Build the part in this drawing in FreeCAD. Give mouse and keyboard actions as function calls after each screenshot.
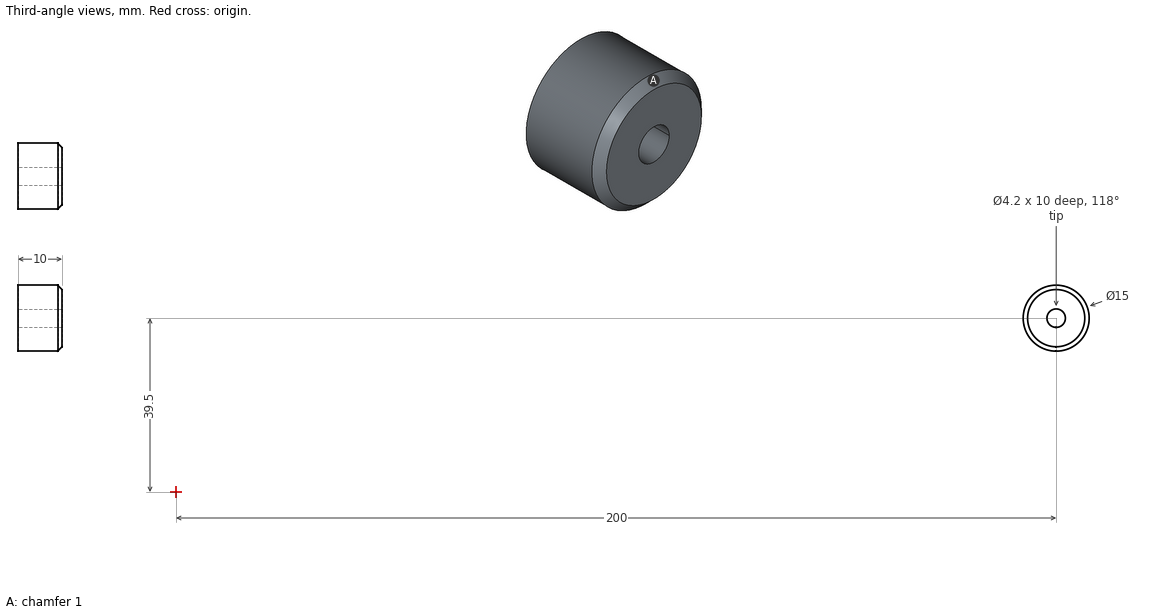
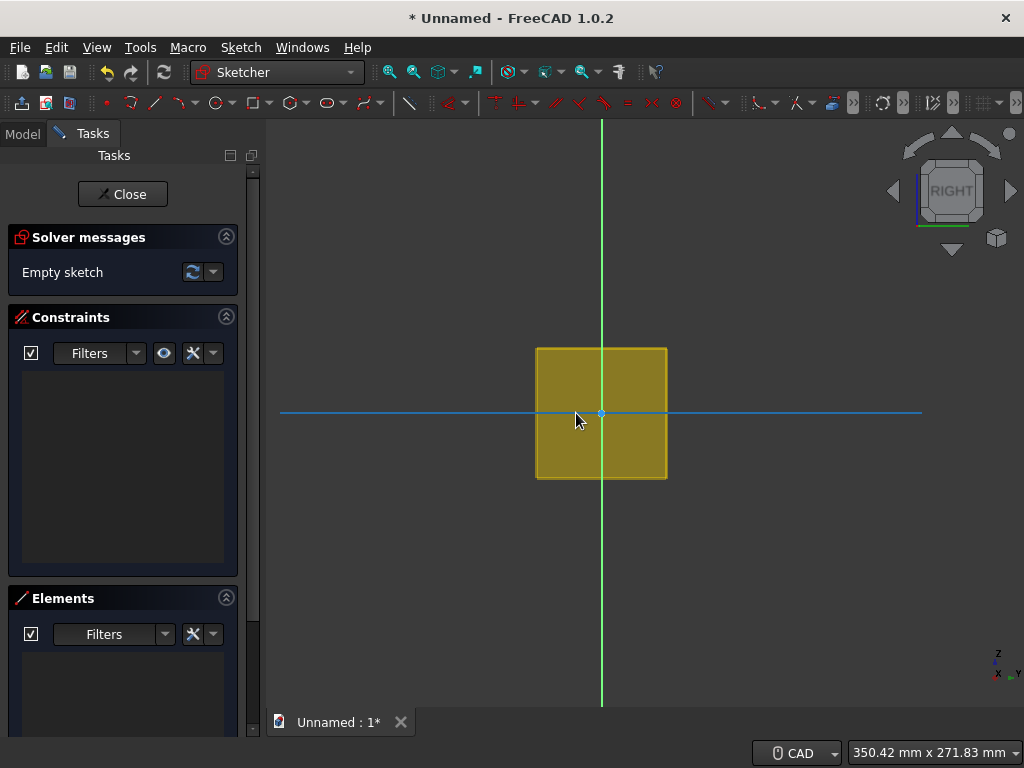
scroll(576, 413, down, 5)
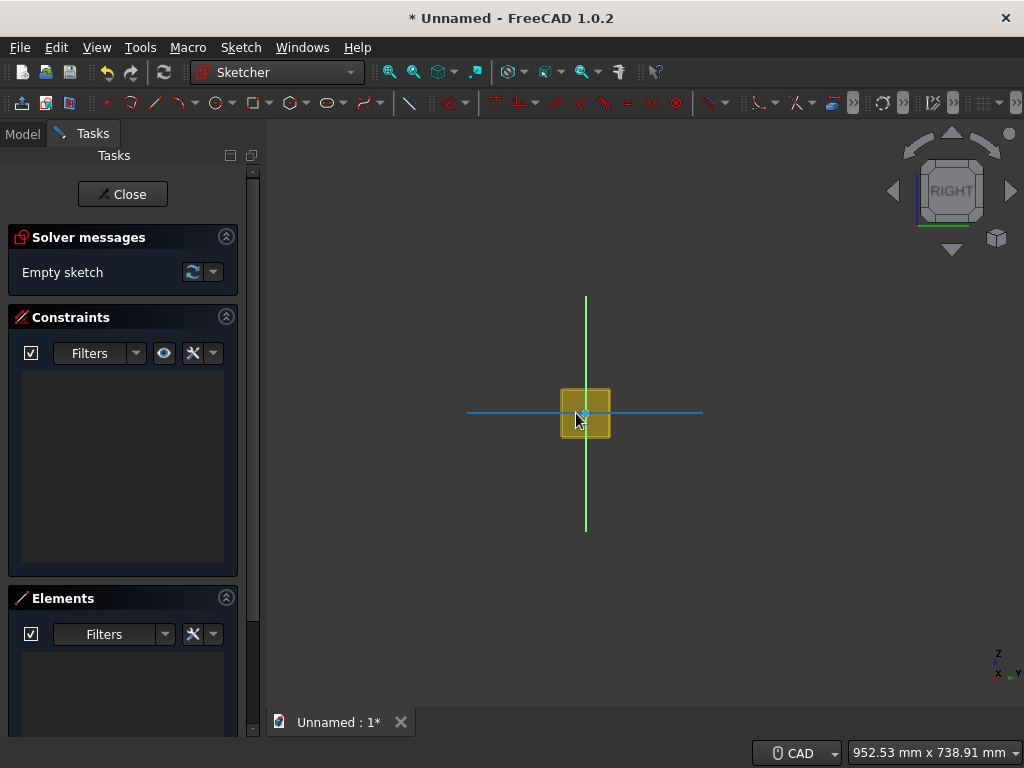
scroll(754, 380, up, 15)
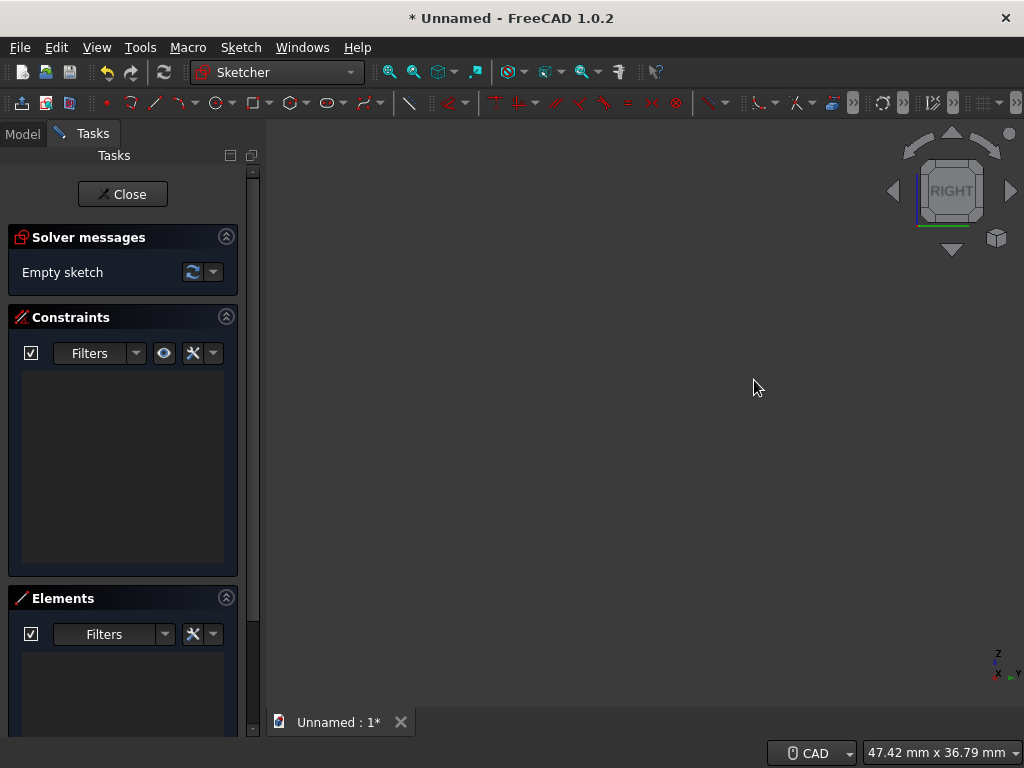
scroll(520, 409, up, 2)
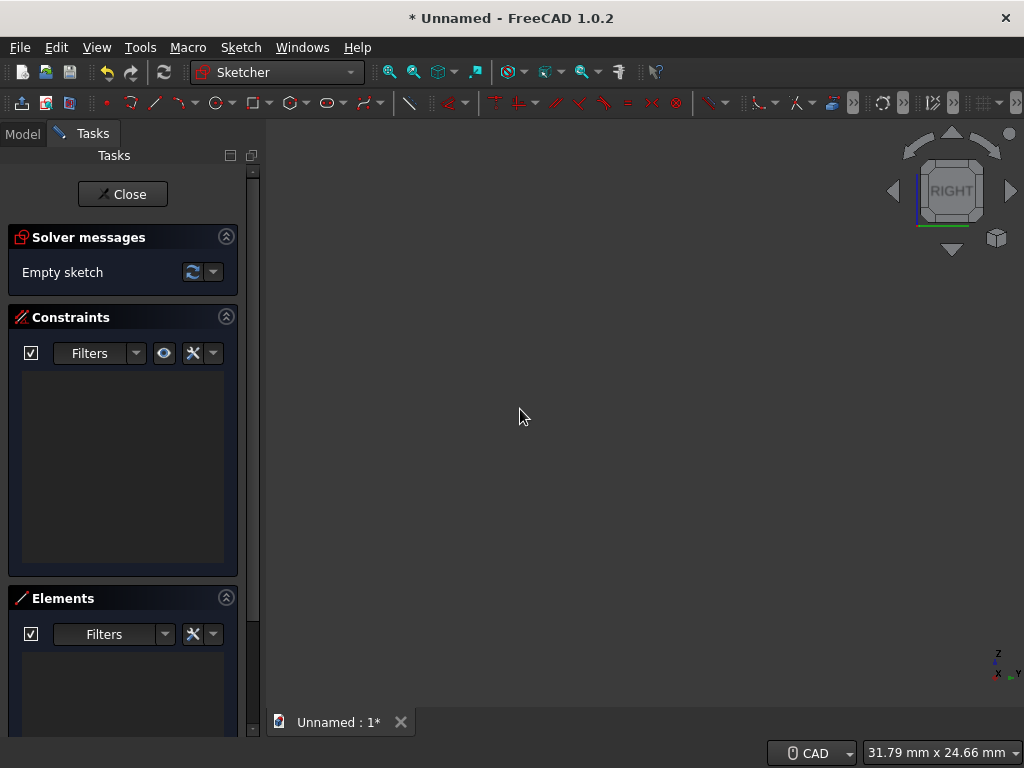
click(216, 104)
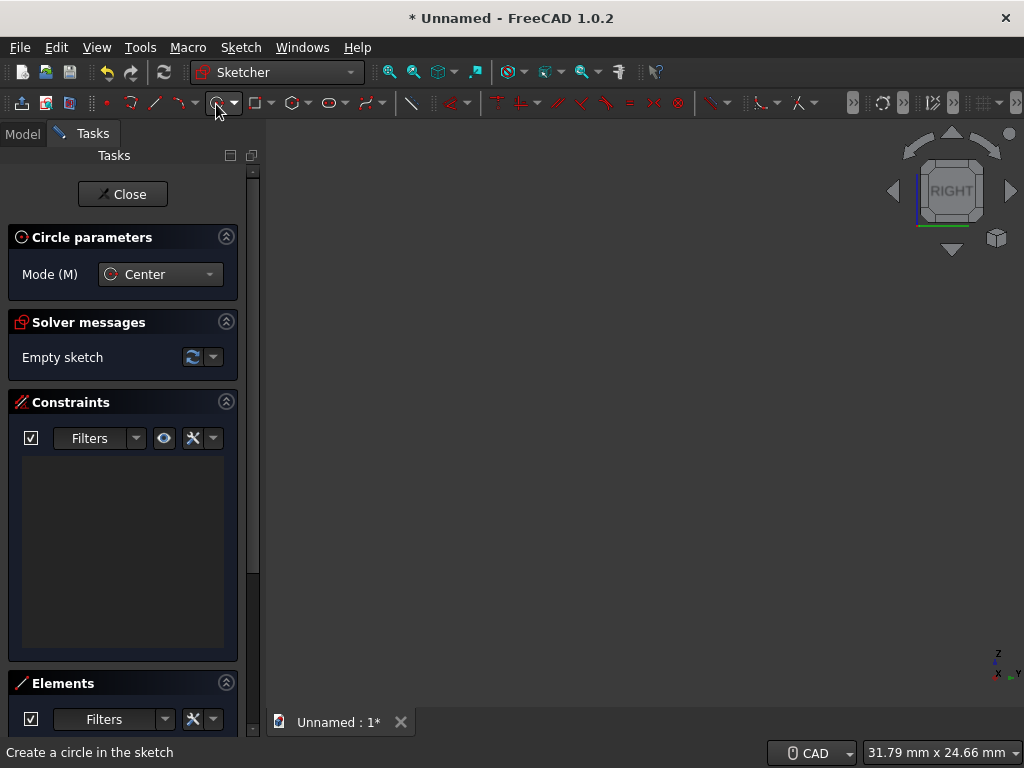
click(576, 413)
move(703, 286)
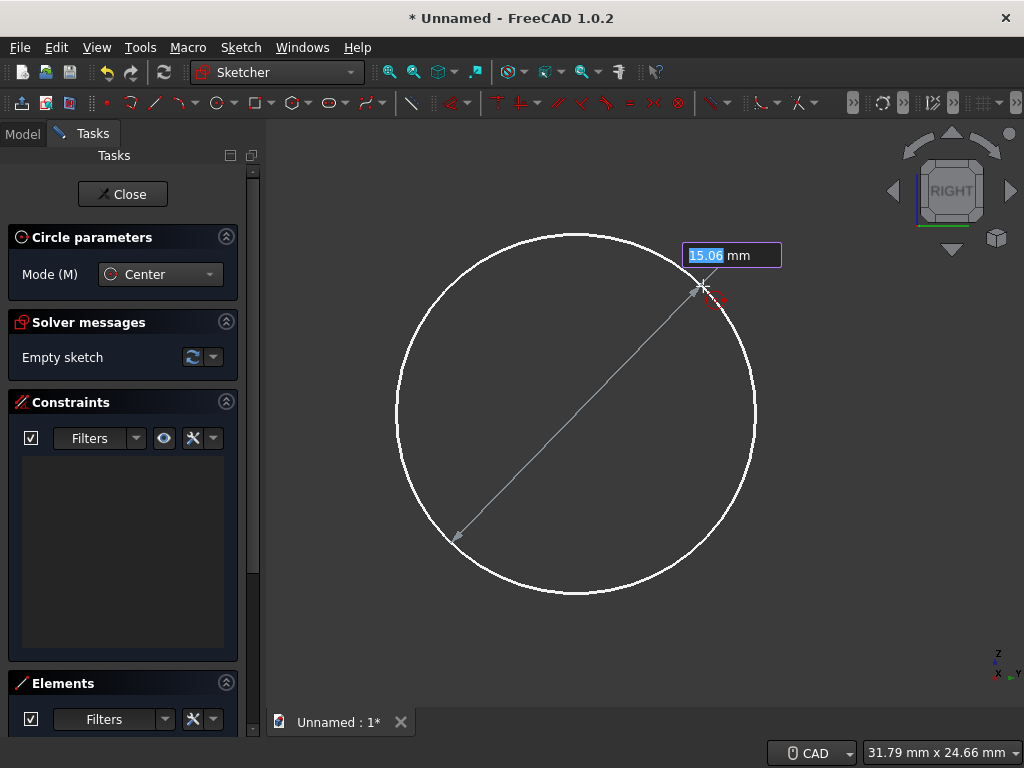
text(15)
key(Return)
key(Escape)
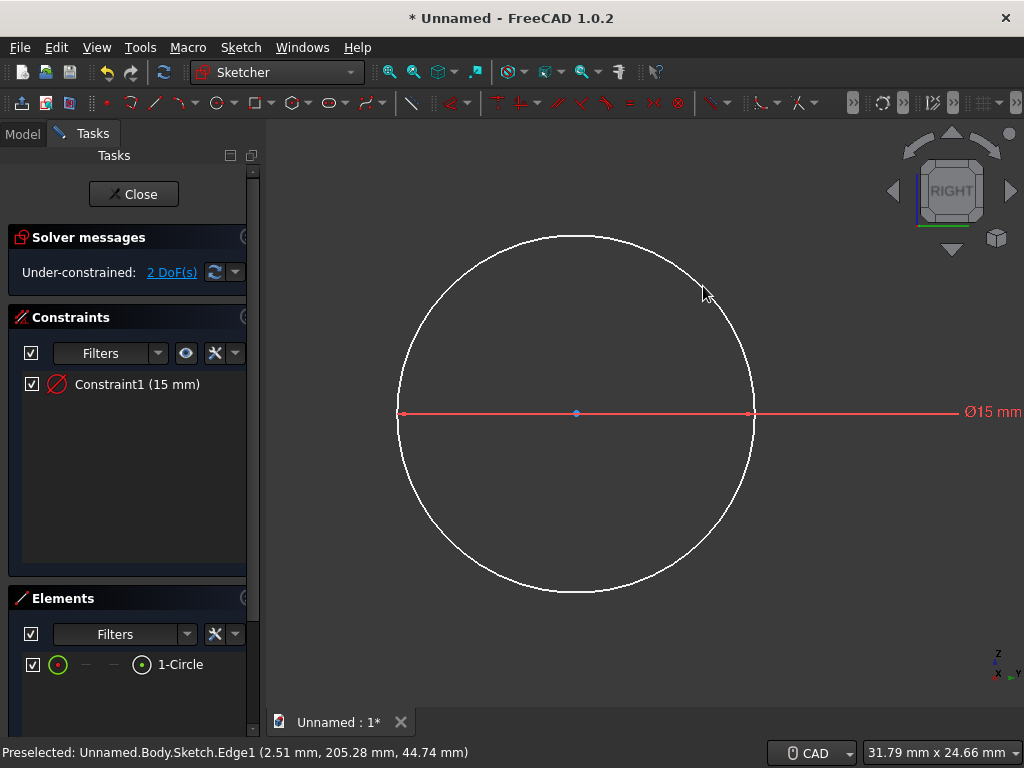
click(450, 104)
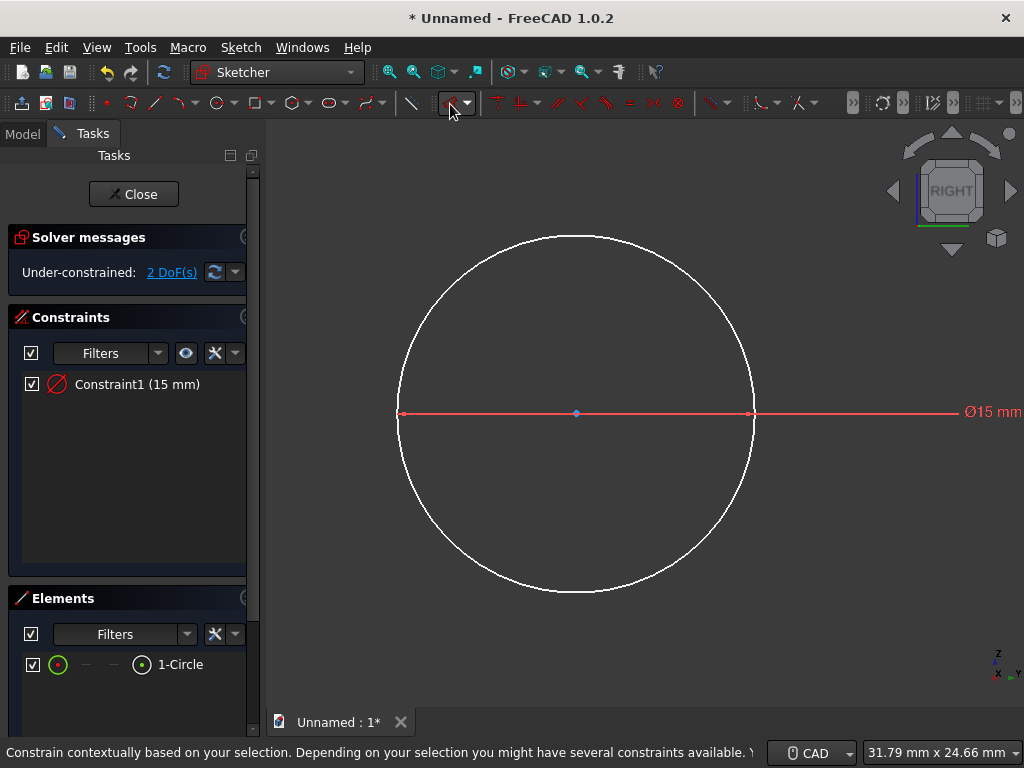
click(576, 414)
click(435, 380)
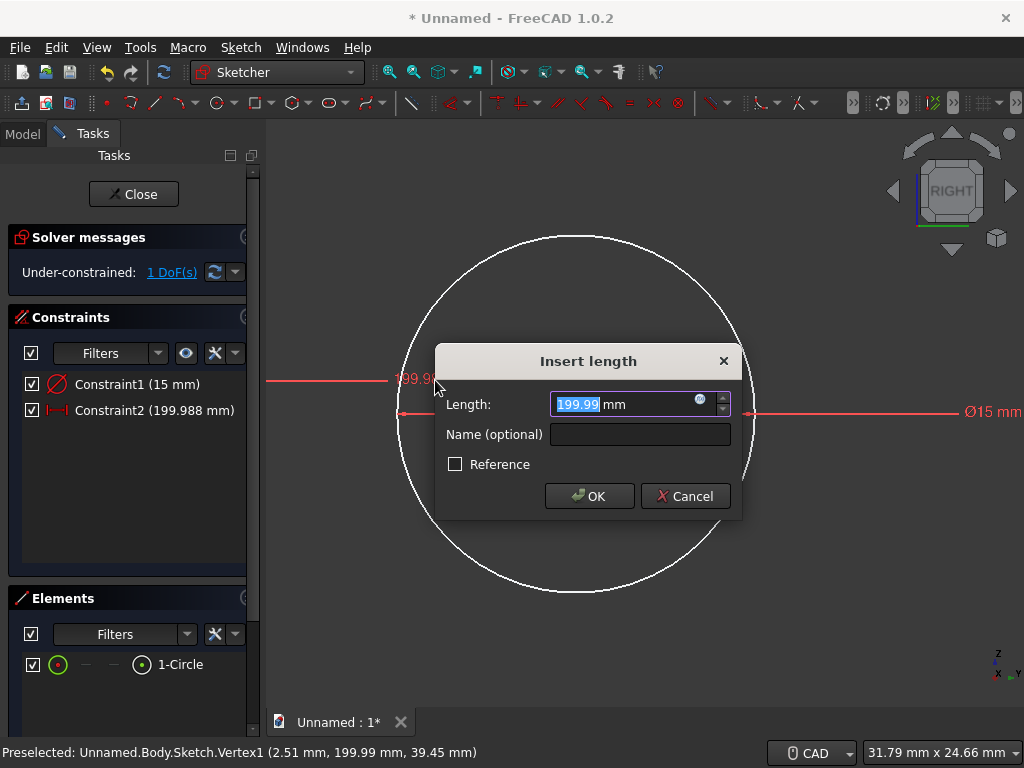
text(200)
key(Return)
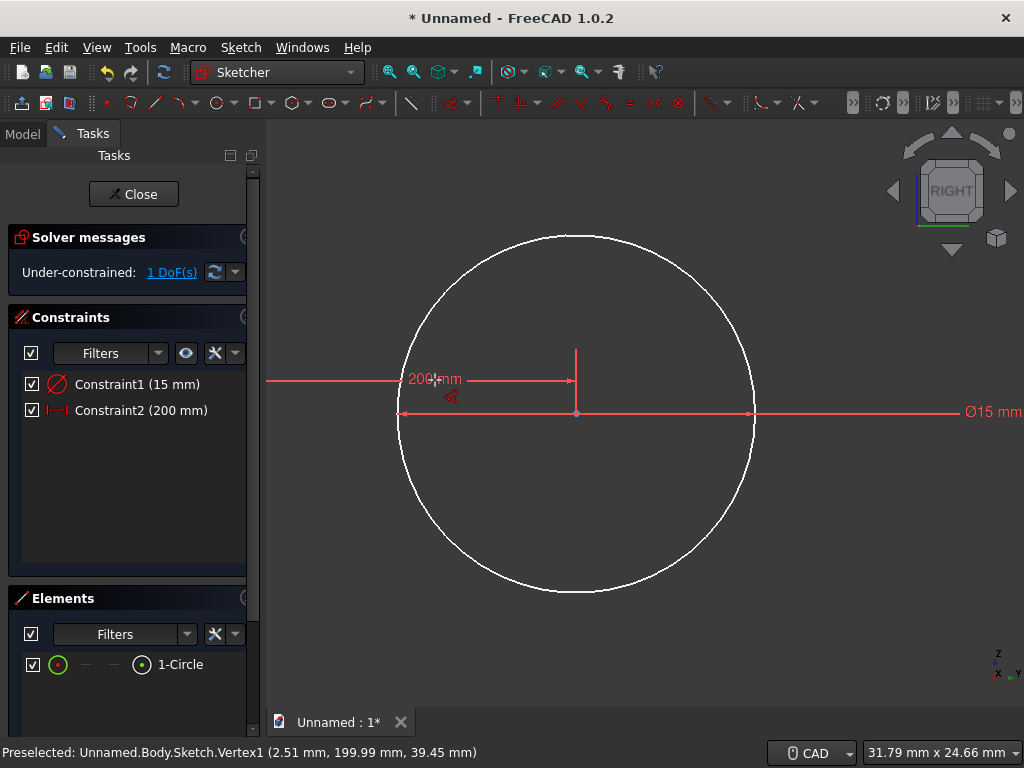
click(576, 414)
click(610, 547)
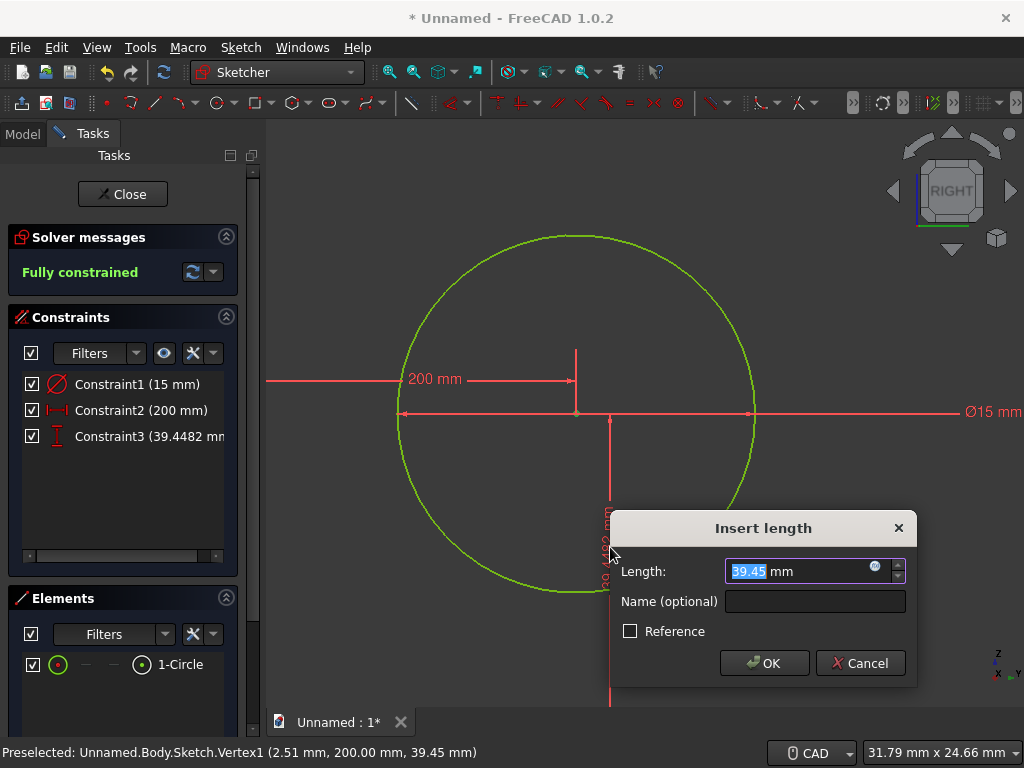
text(39.5)
key(Return)
key(Escape)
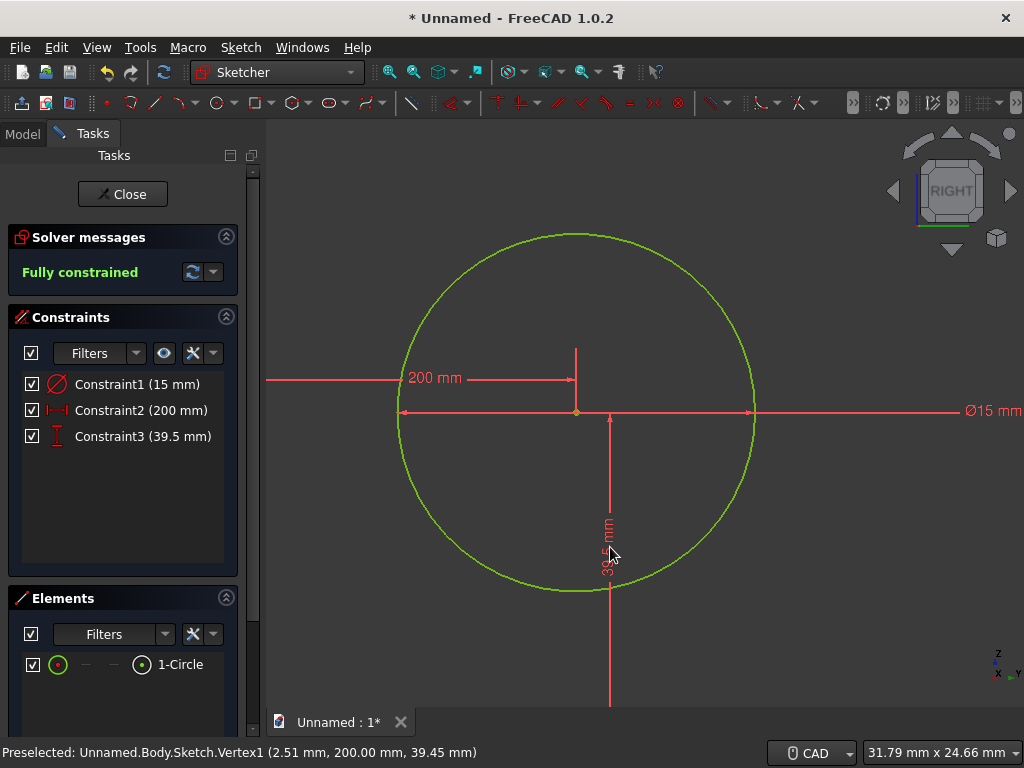
click(123, 194)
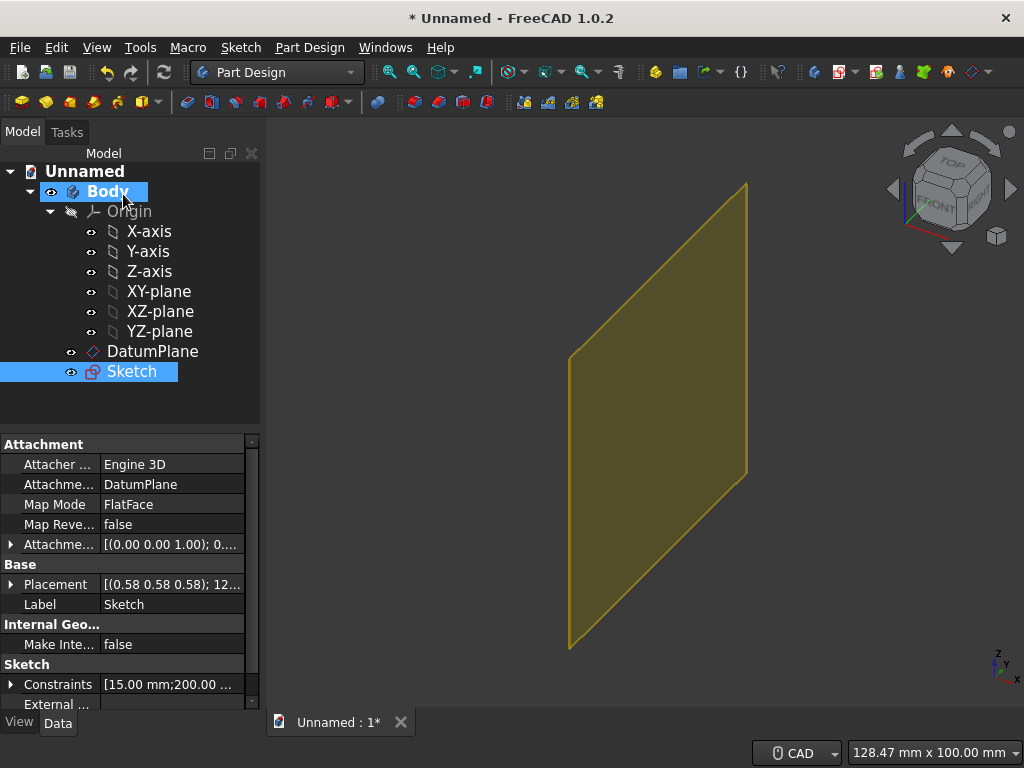
click(22, 102)